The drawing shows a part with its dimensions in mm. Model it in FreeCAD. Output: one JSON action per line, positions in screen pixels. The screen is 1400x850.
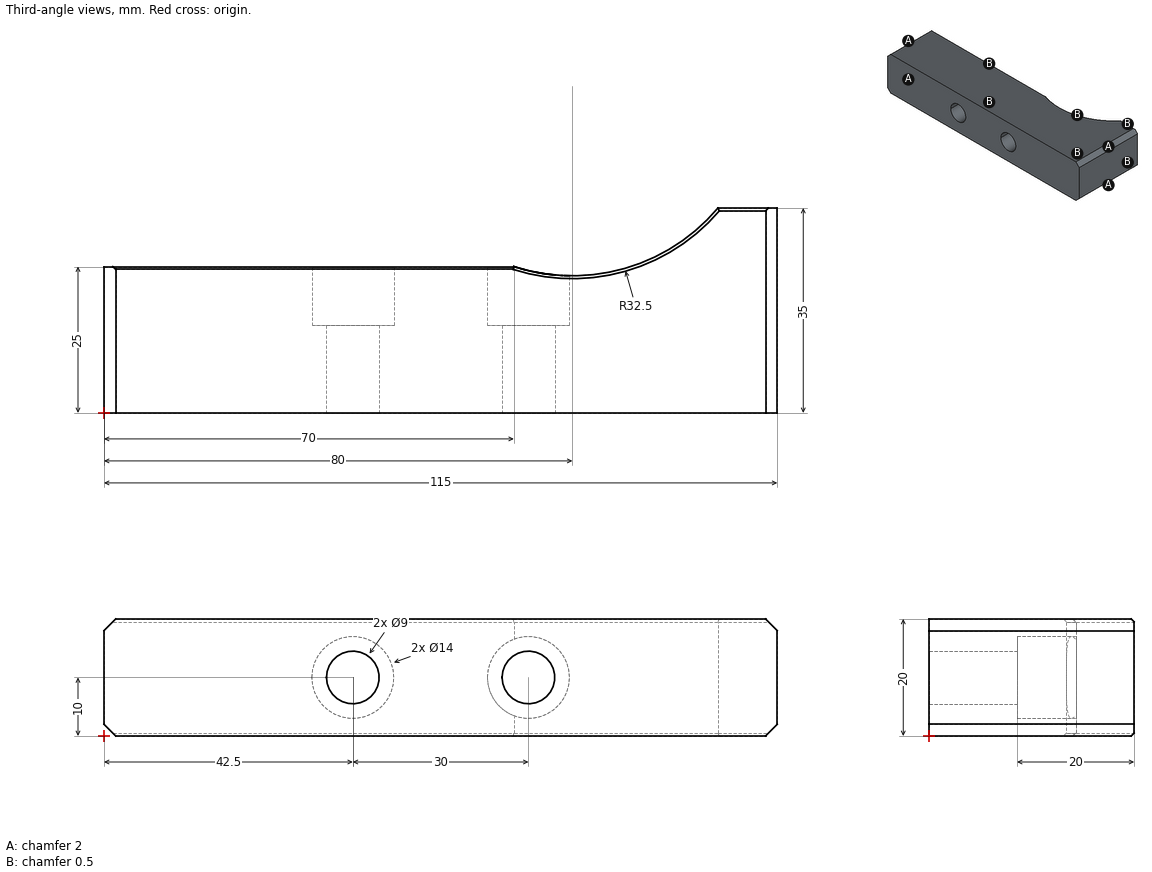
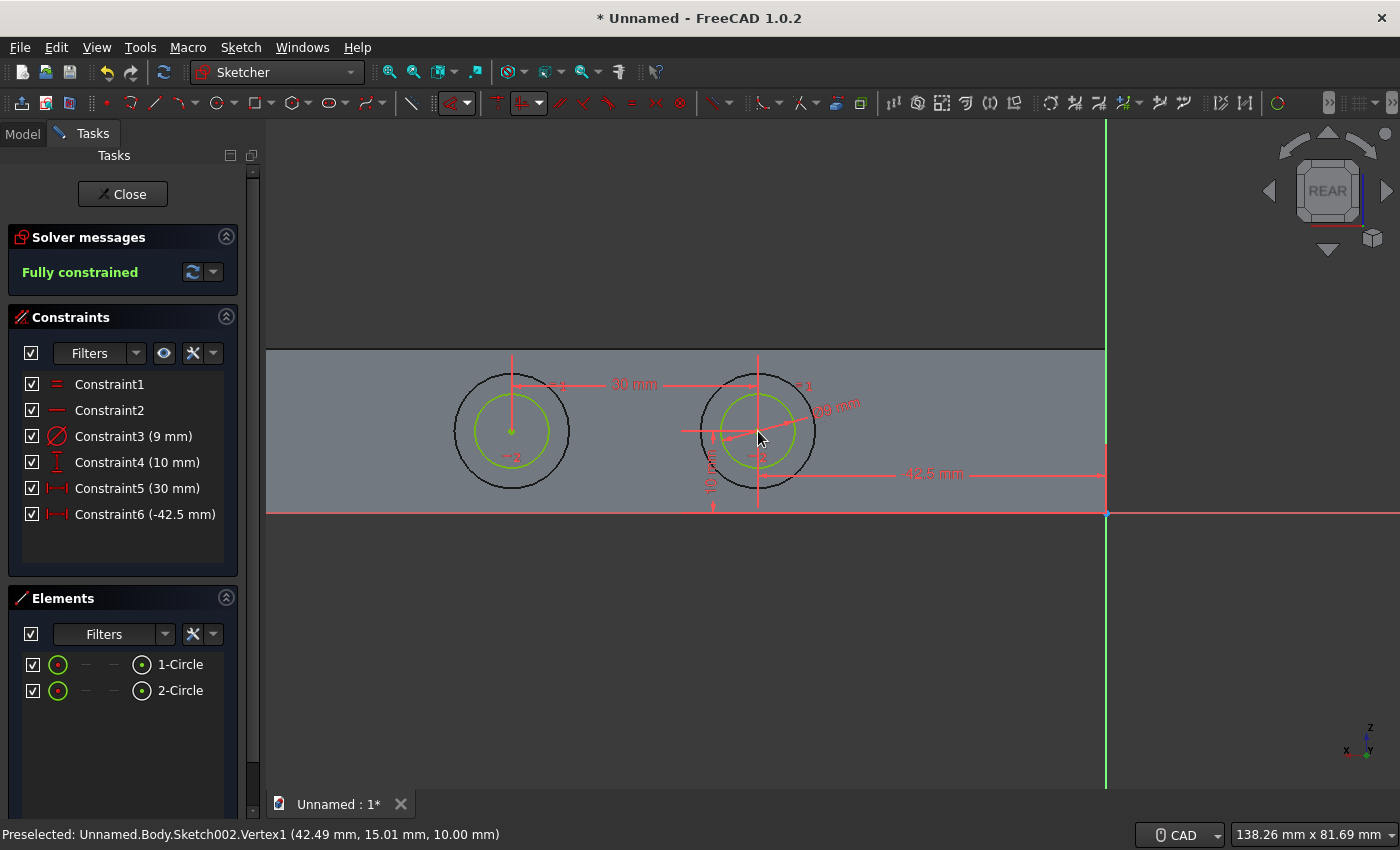
{"action": "left_click", "coordinate": [123, 194]}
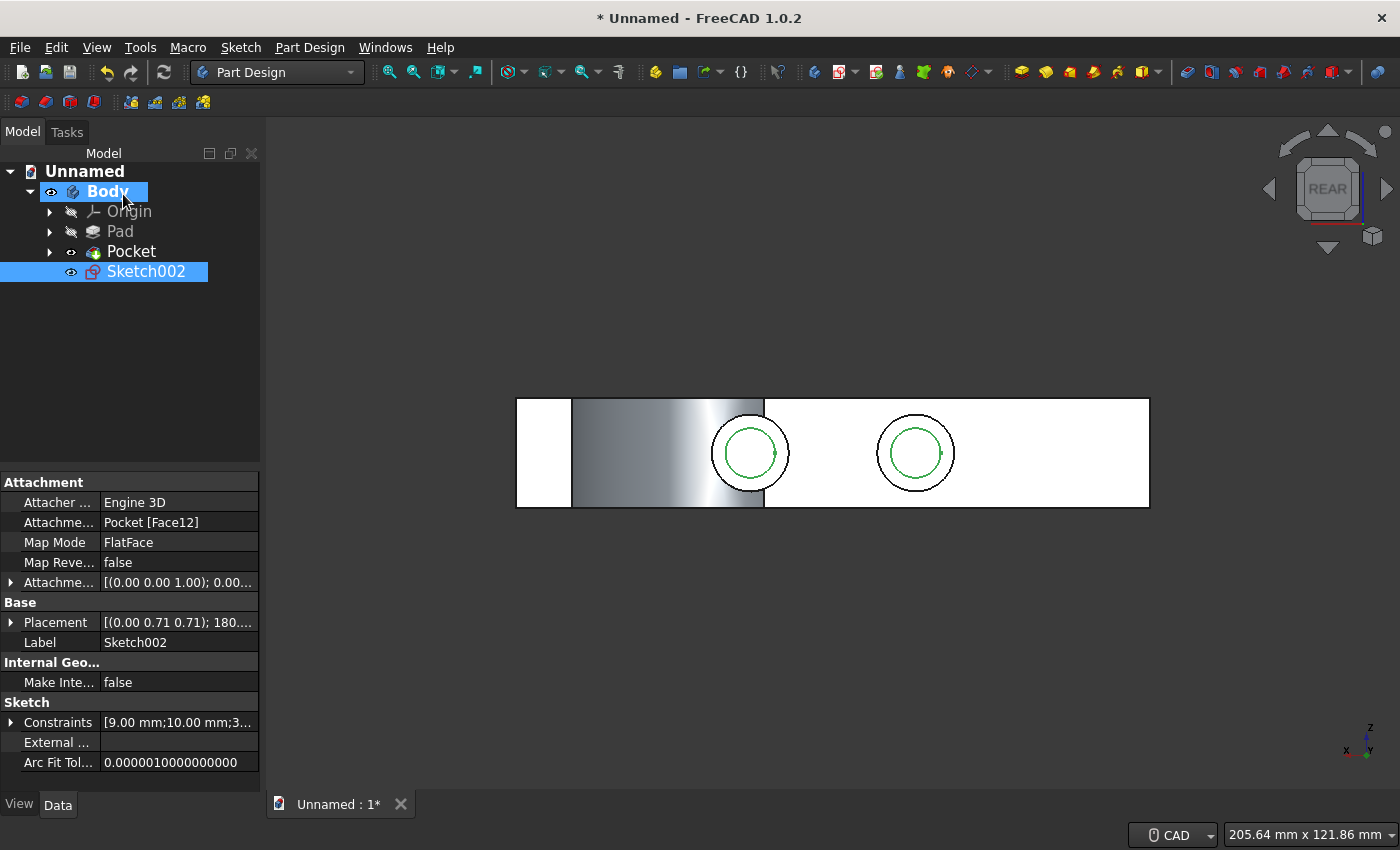
{"action": "left_click", "coordinate": [1188, 72]}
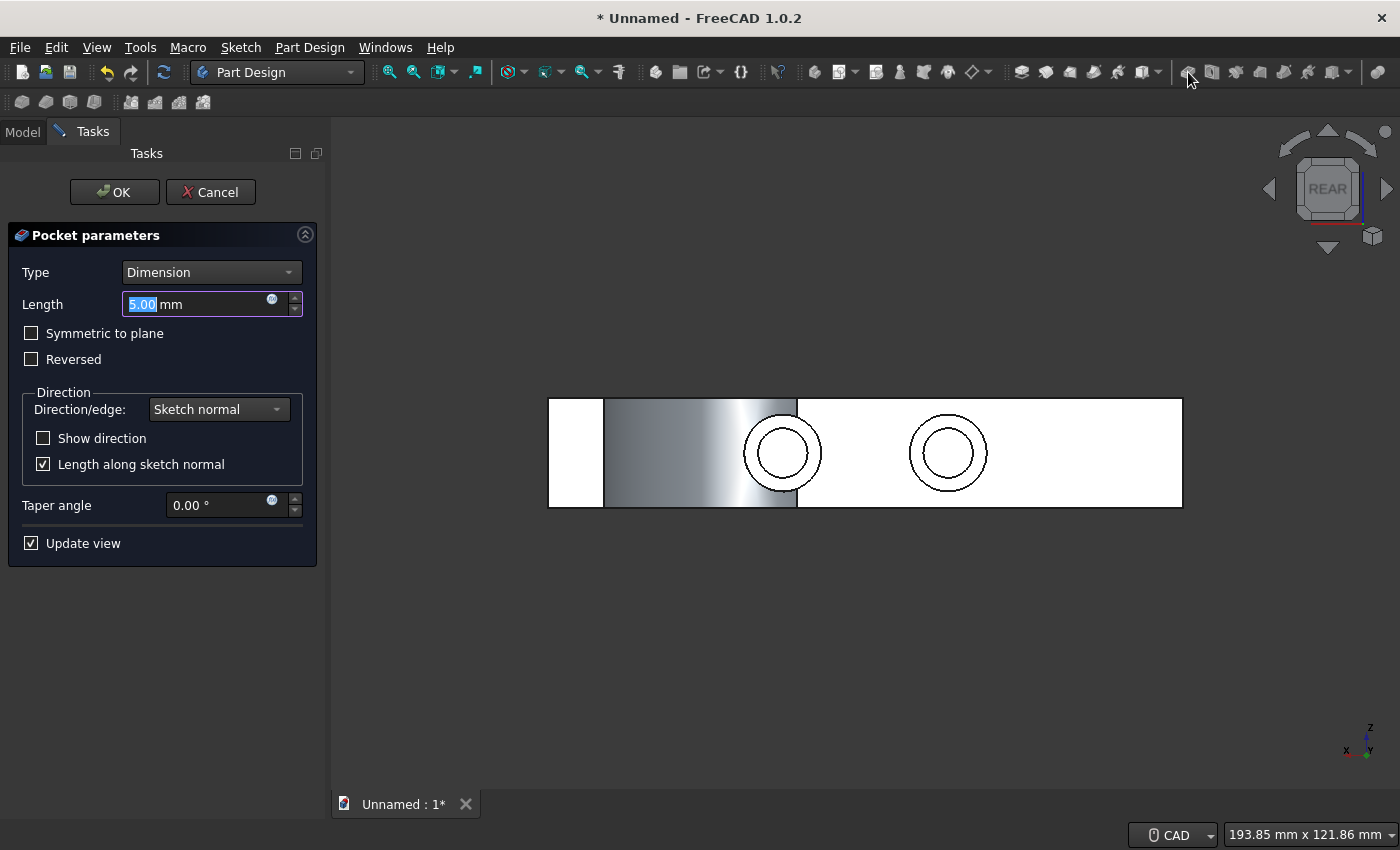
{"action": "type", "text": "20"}
{"action": "key", "text": "Tab"}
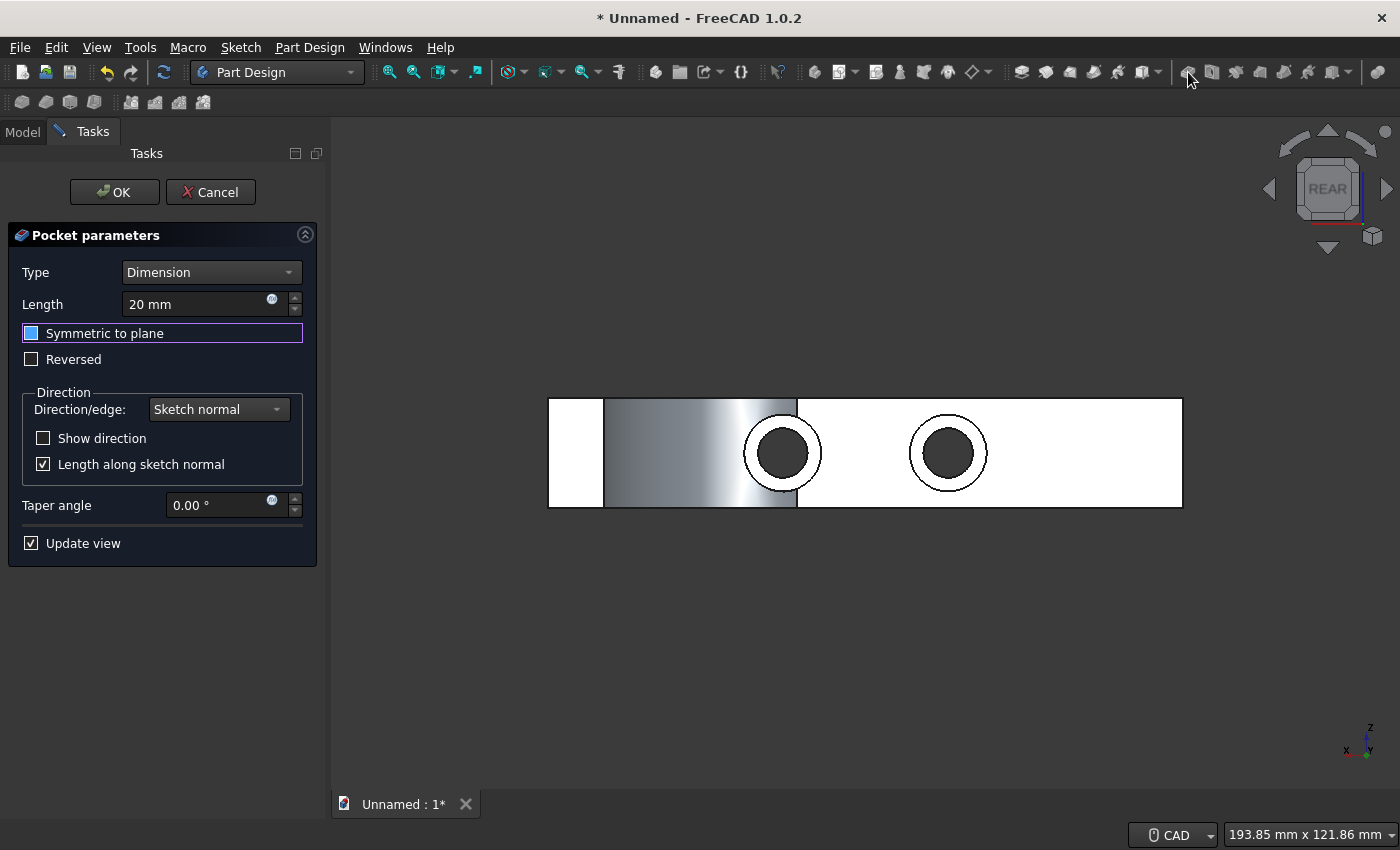
{"action": "left_click", "coordinate": [115, 192]}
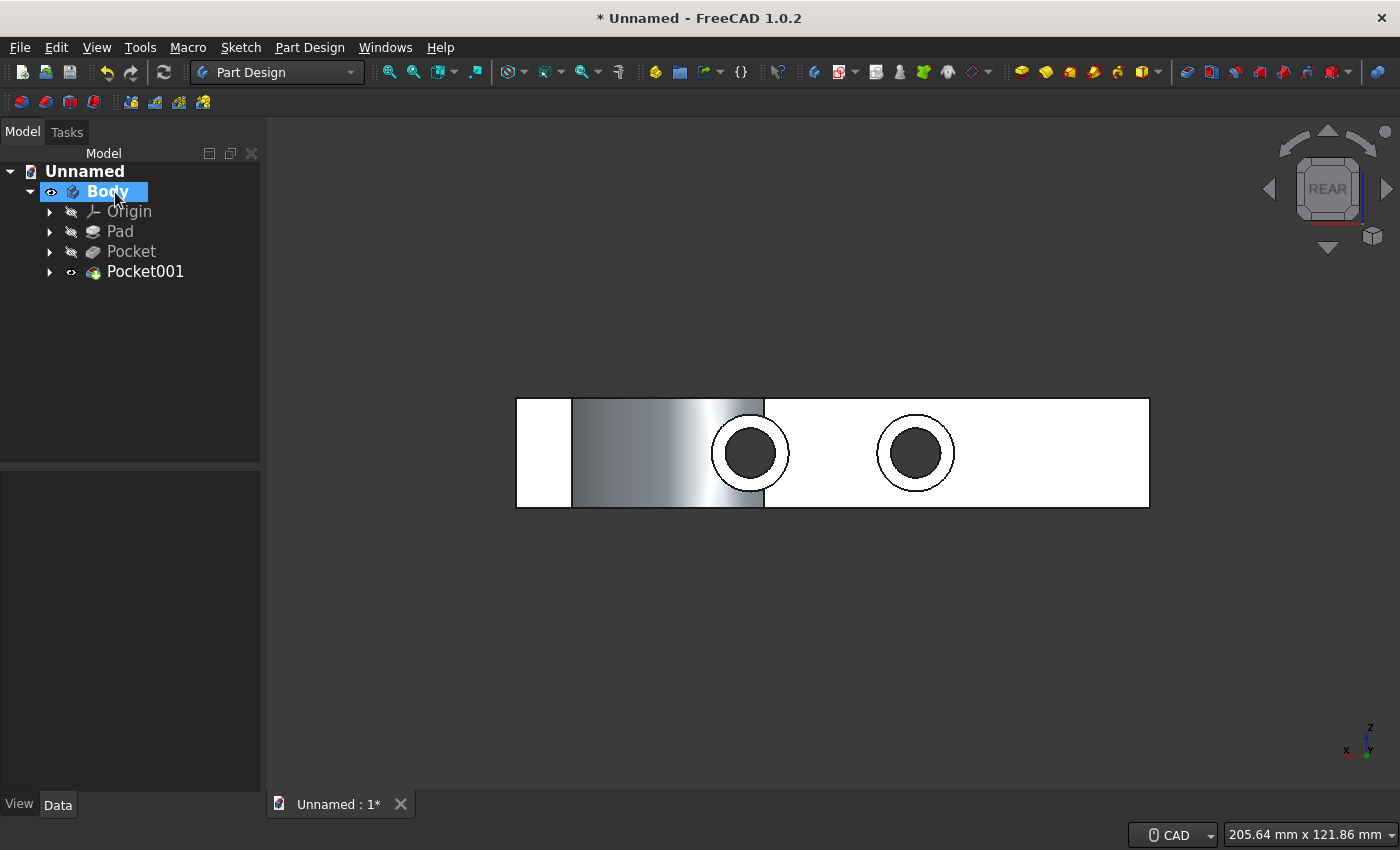
{"action": "key", "text": "0"}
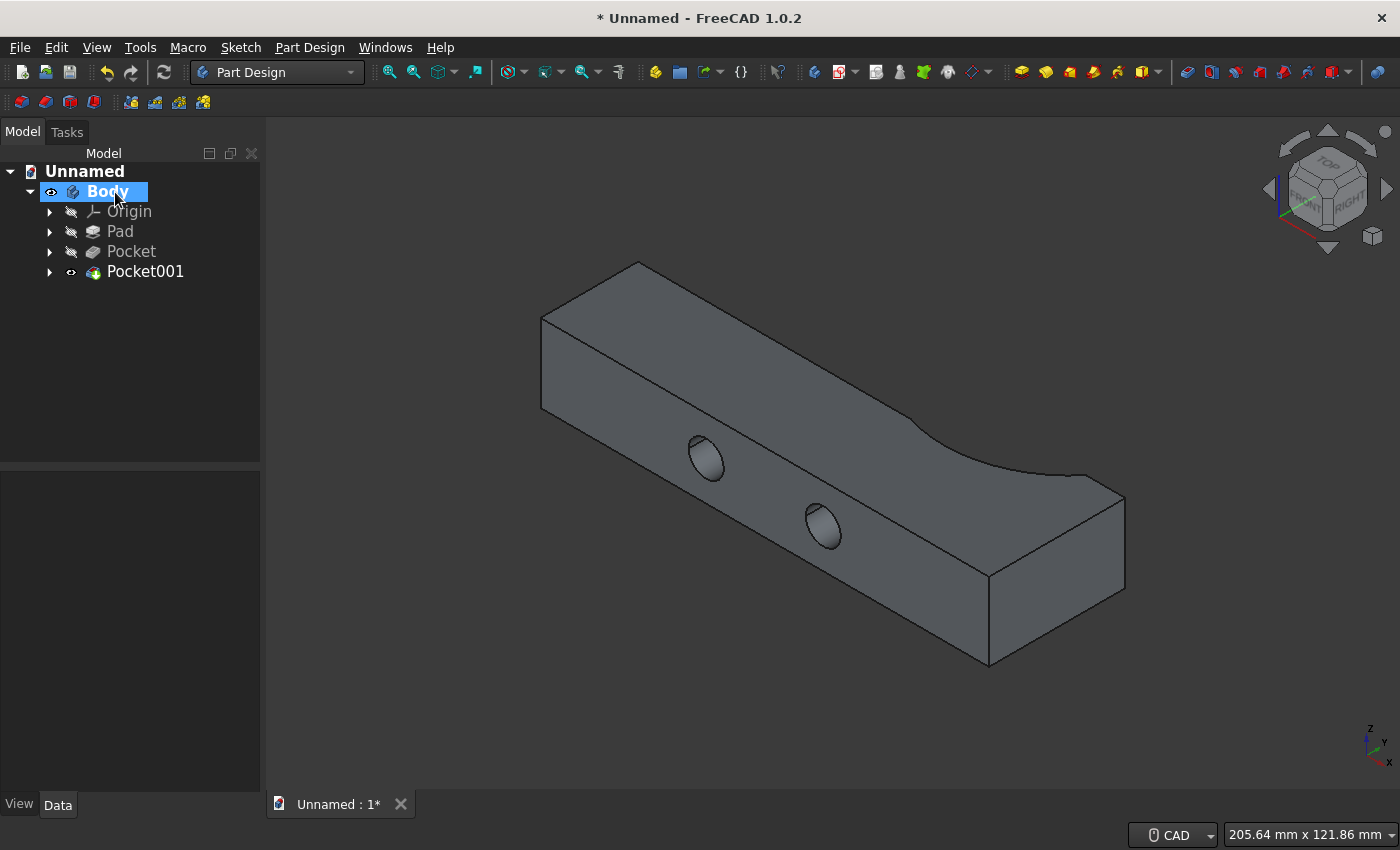
{"action": "left_click", "coordinate": [1057, 536]}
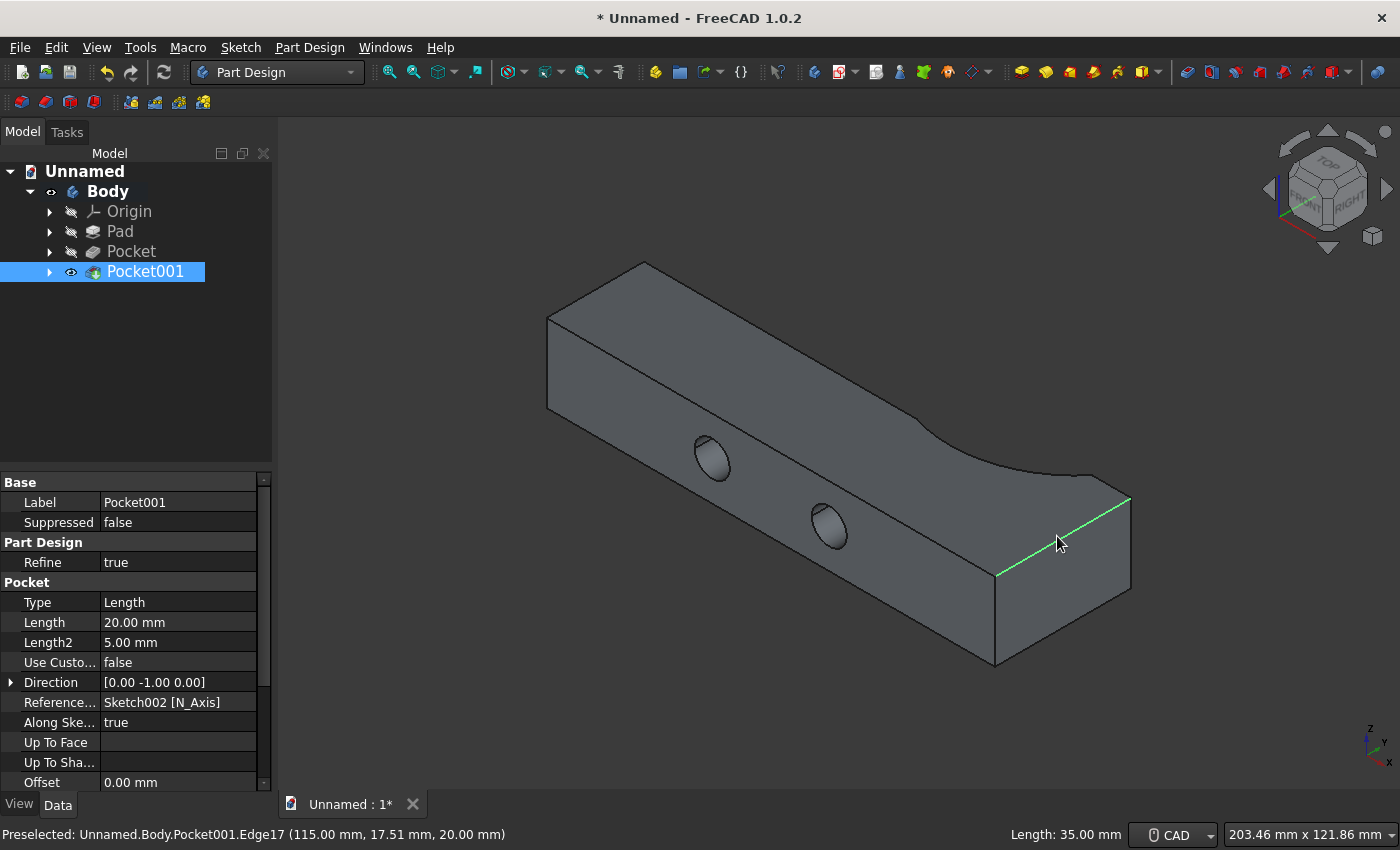
{"action": "key", "text": "2"}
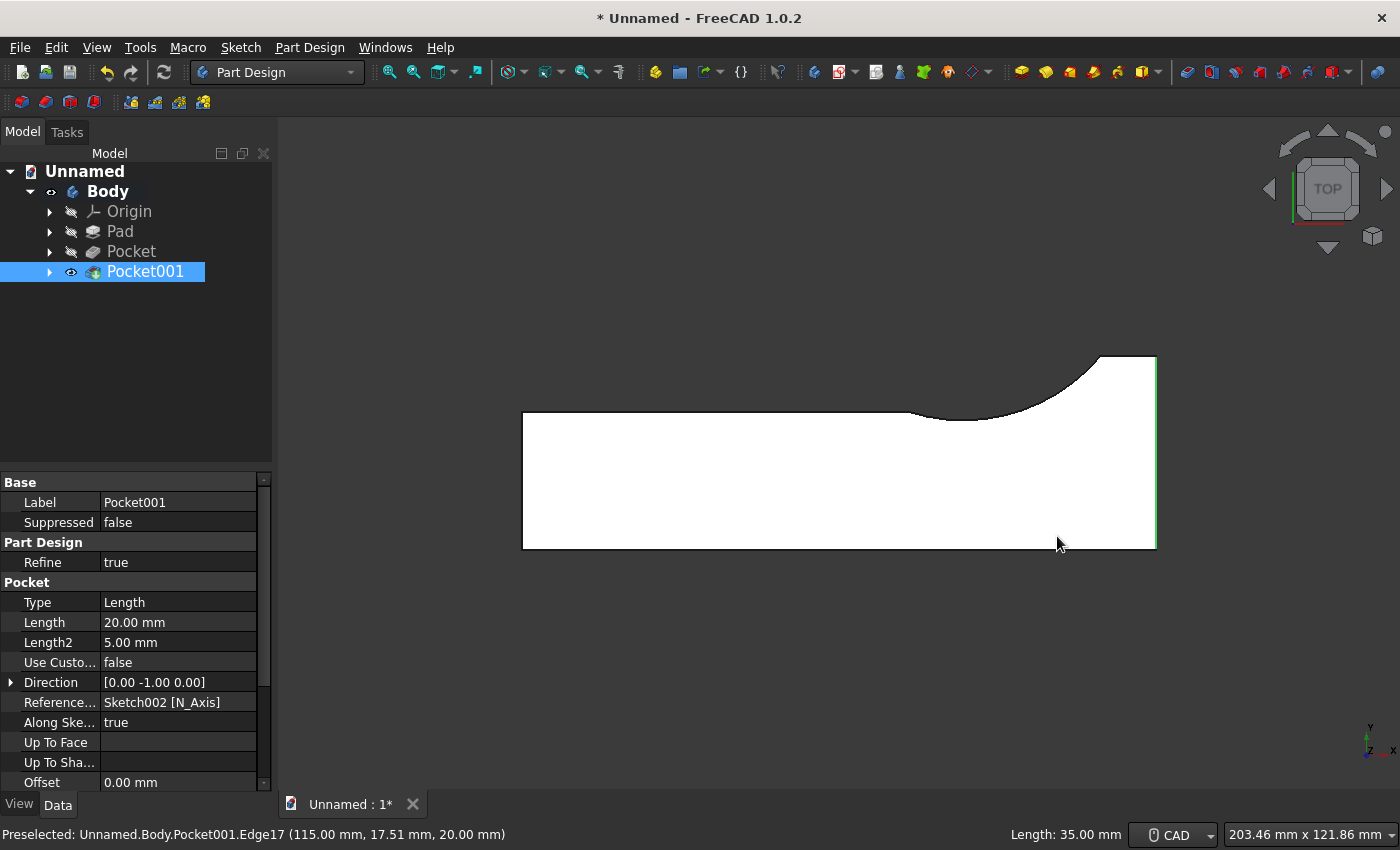
{"action": "left_click", "coordinate": [522, 480], "text": "ctrl"}